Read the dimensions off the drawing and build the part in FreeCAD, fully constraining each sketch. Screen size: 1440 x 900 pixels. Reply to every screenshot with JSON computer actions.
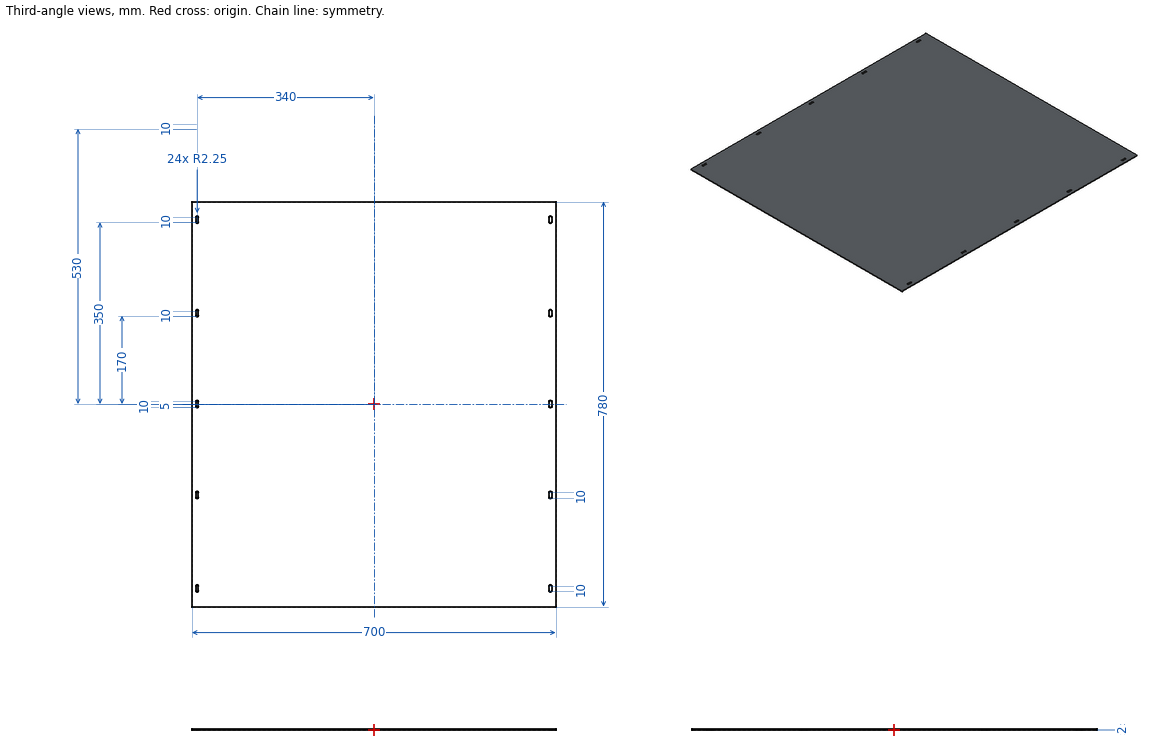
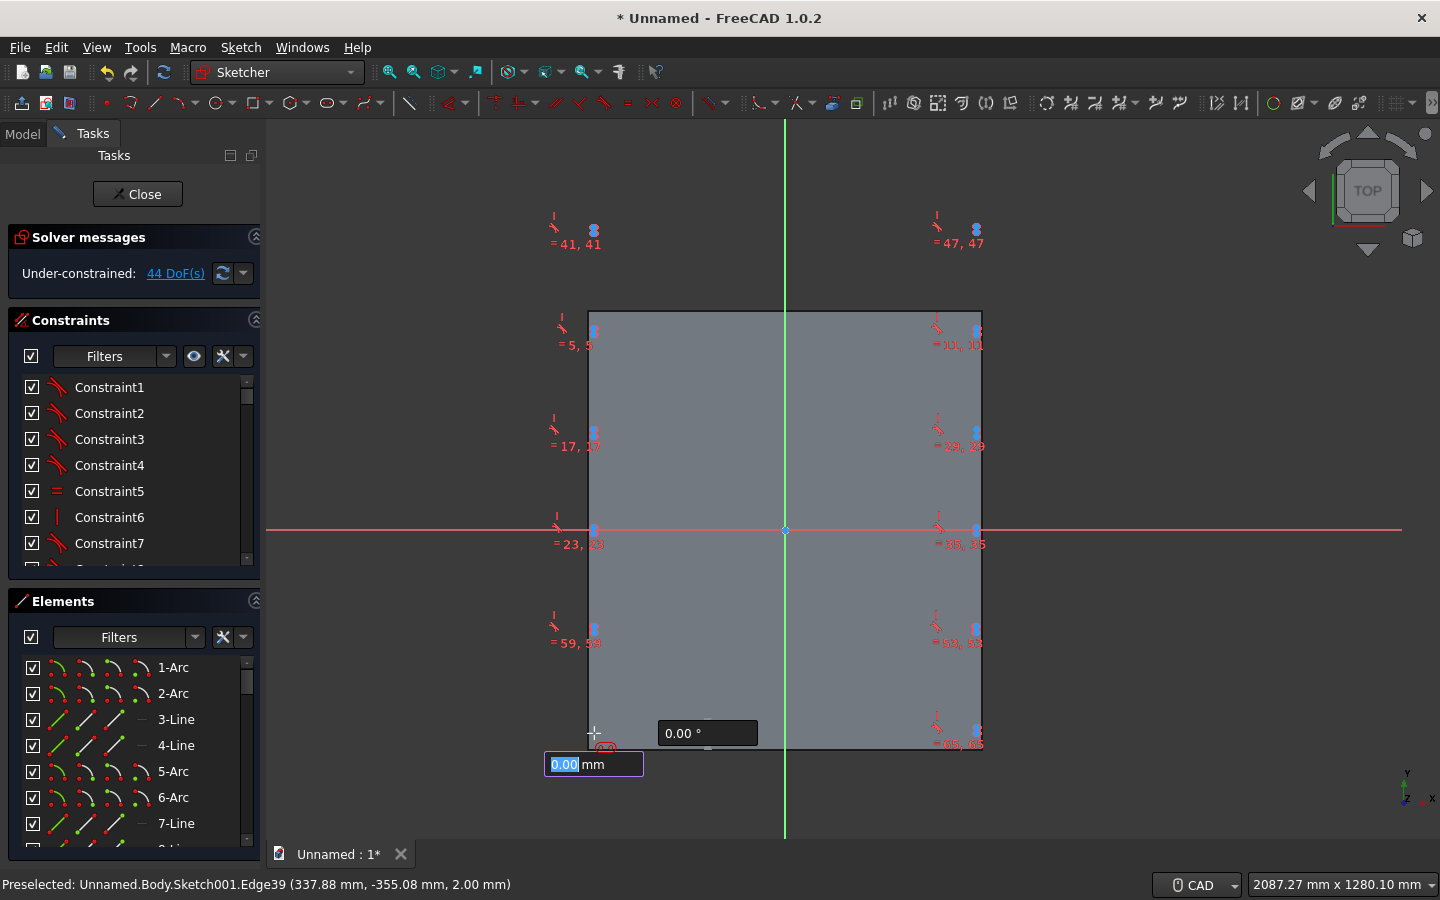
{"action": "scroll", "coordinate": [594, 727], "scroll_direction": "up", "scroll_amount": 6}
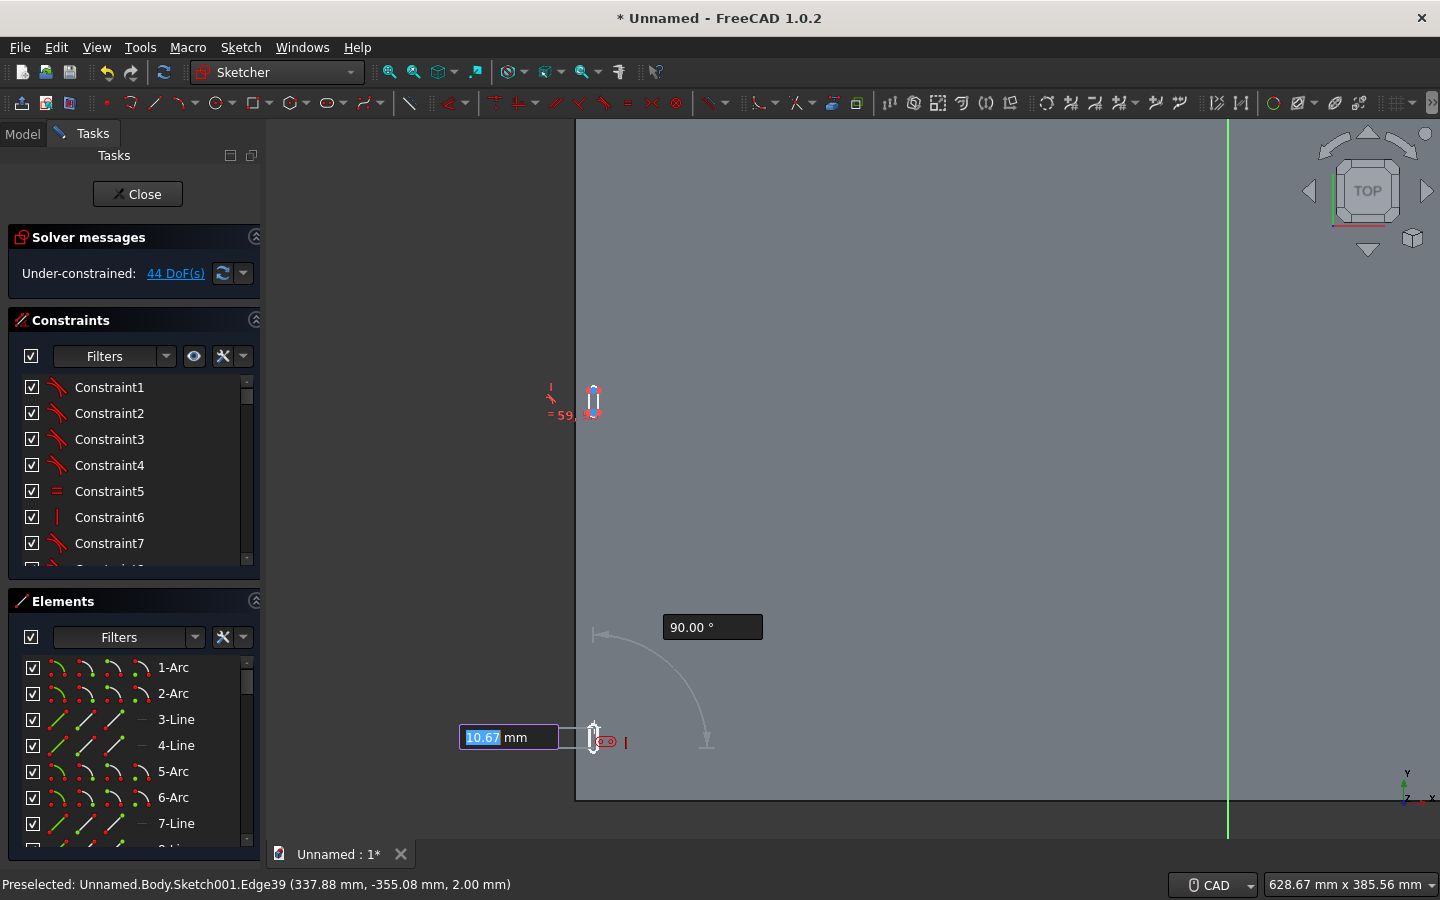
{"action": "left_click", "coordinate": [593, 726]}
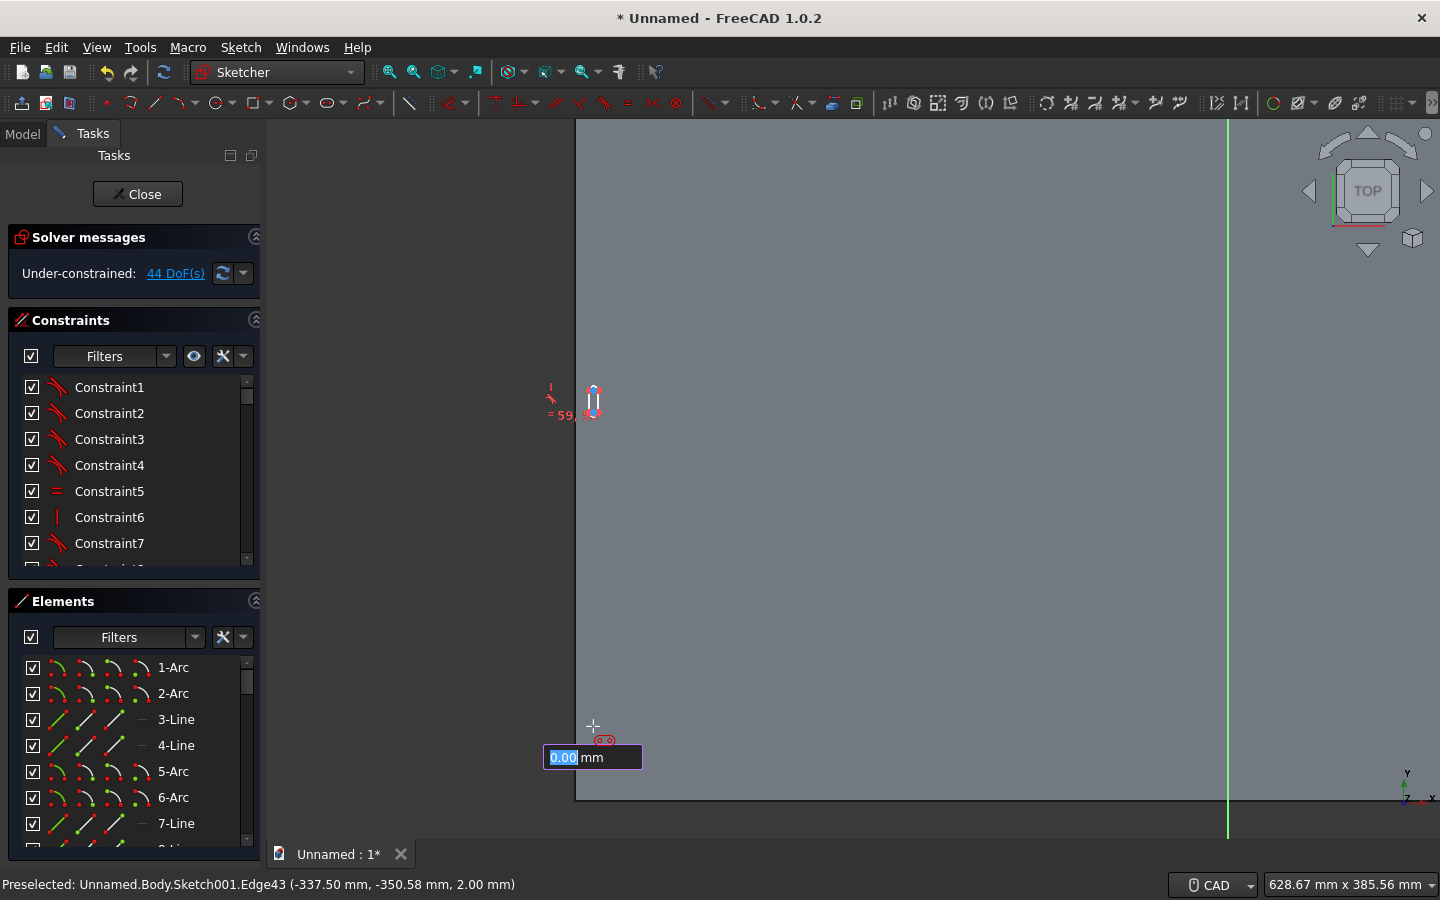
{"action": "scroll", "coordinate": [598, 735], "scroll_direction": "up", "scroll_amount": 7}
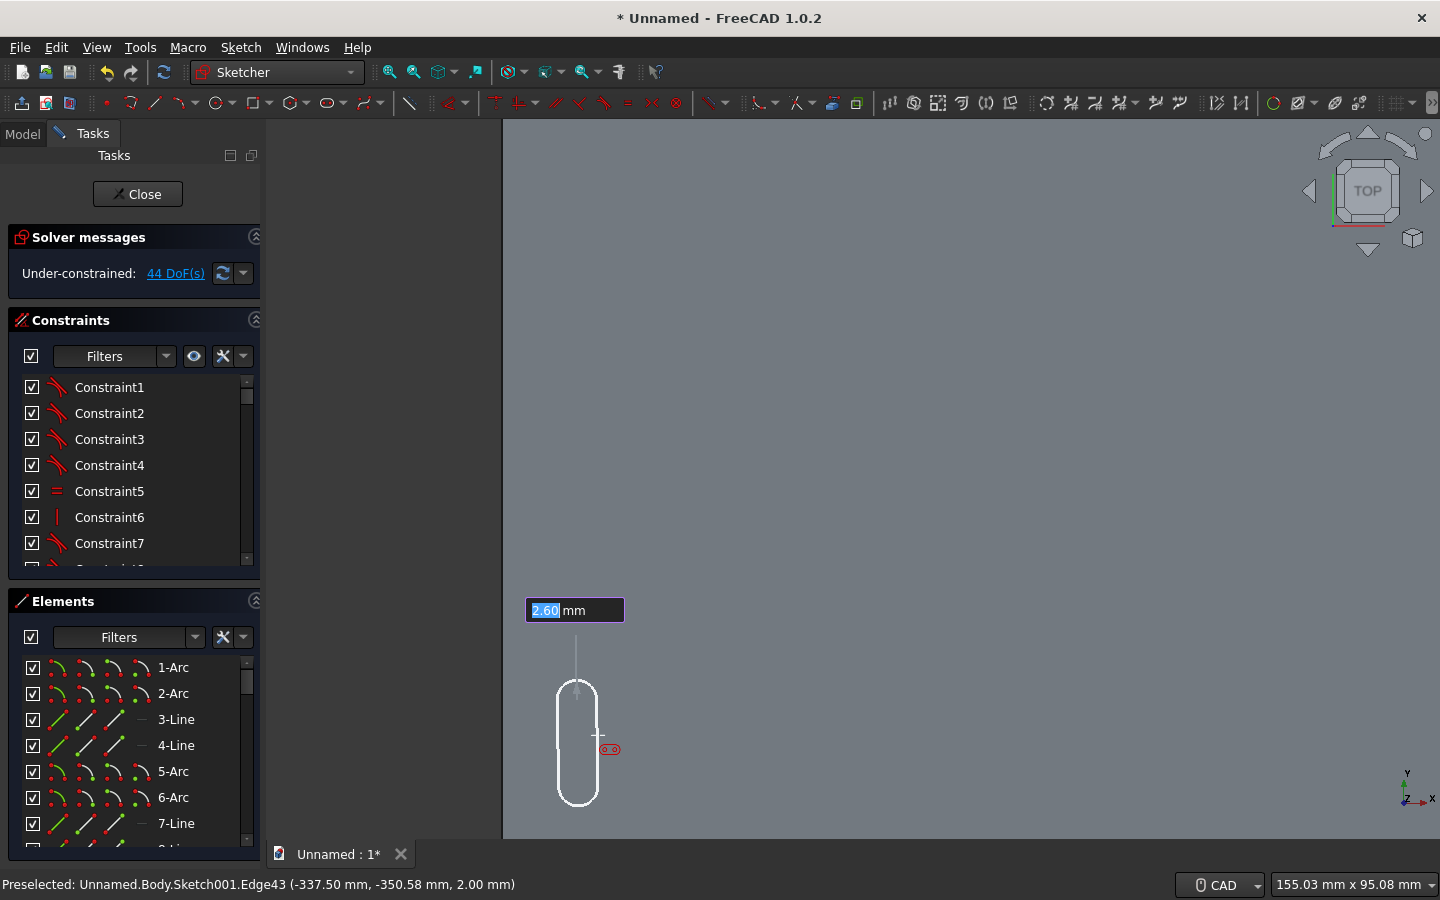
{"action": "left_click", "coordinate": [595, 734]}
{"action": "key", "text": "Escape"}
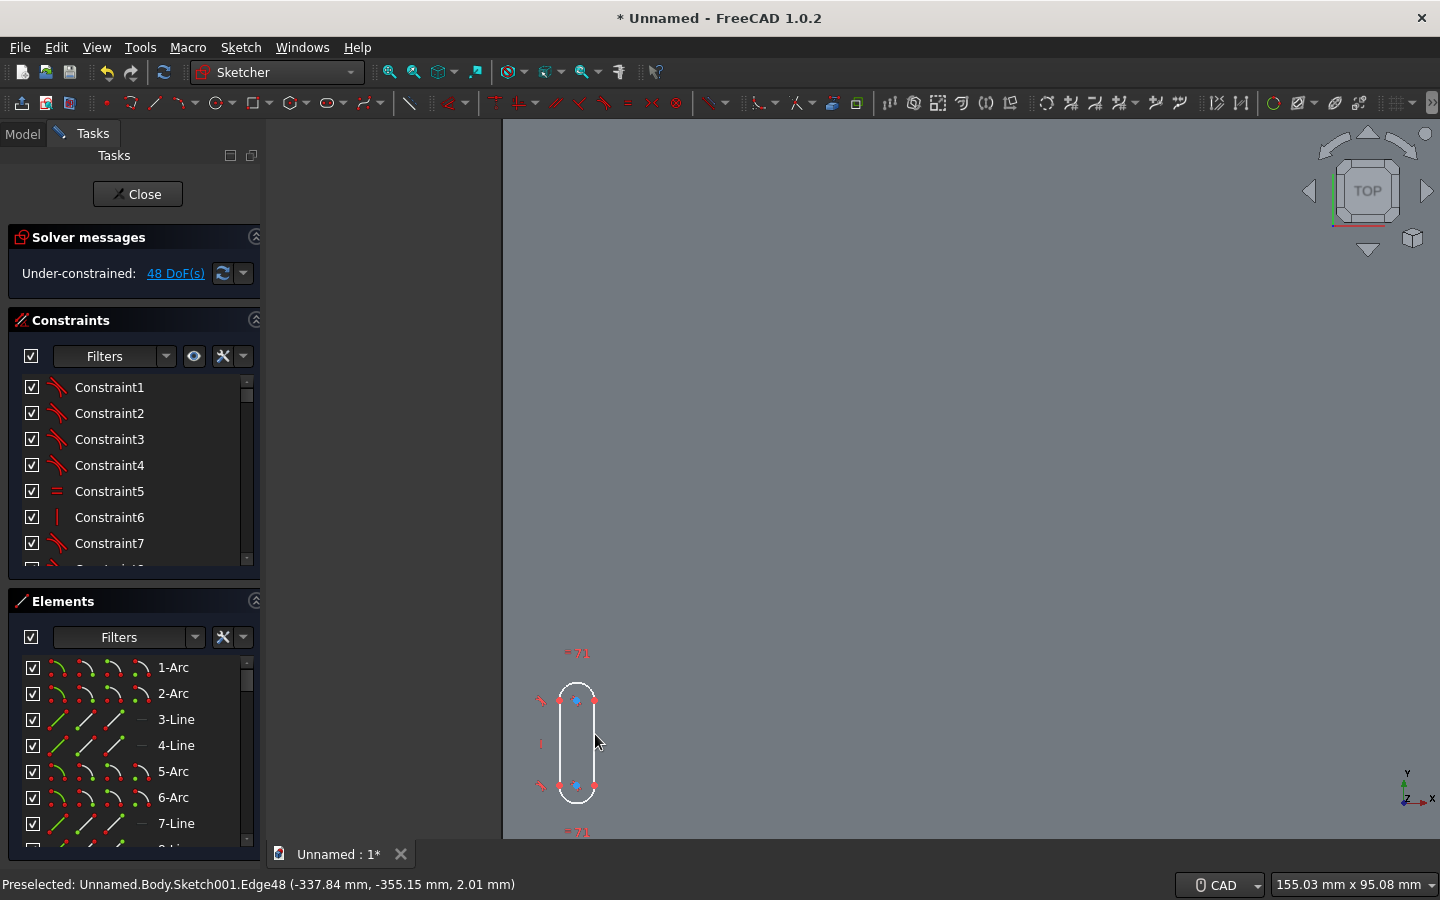
{"action": "scroll", "coordinate": [594, 729], "scroll_direction": "down", "scroll_amount": 13}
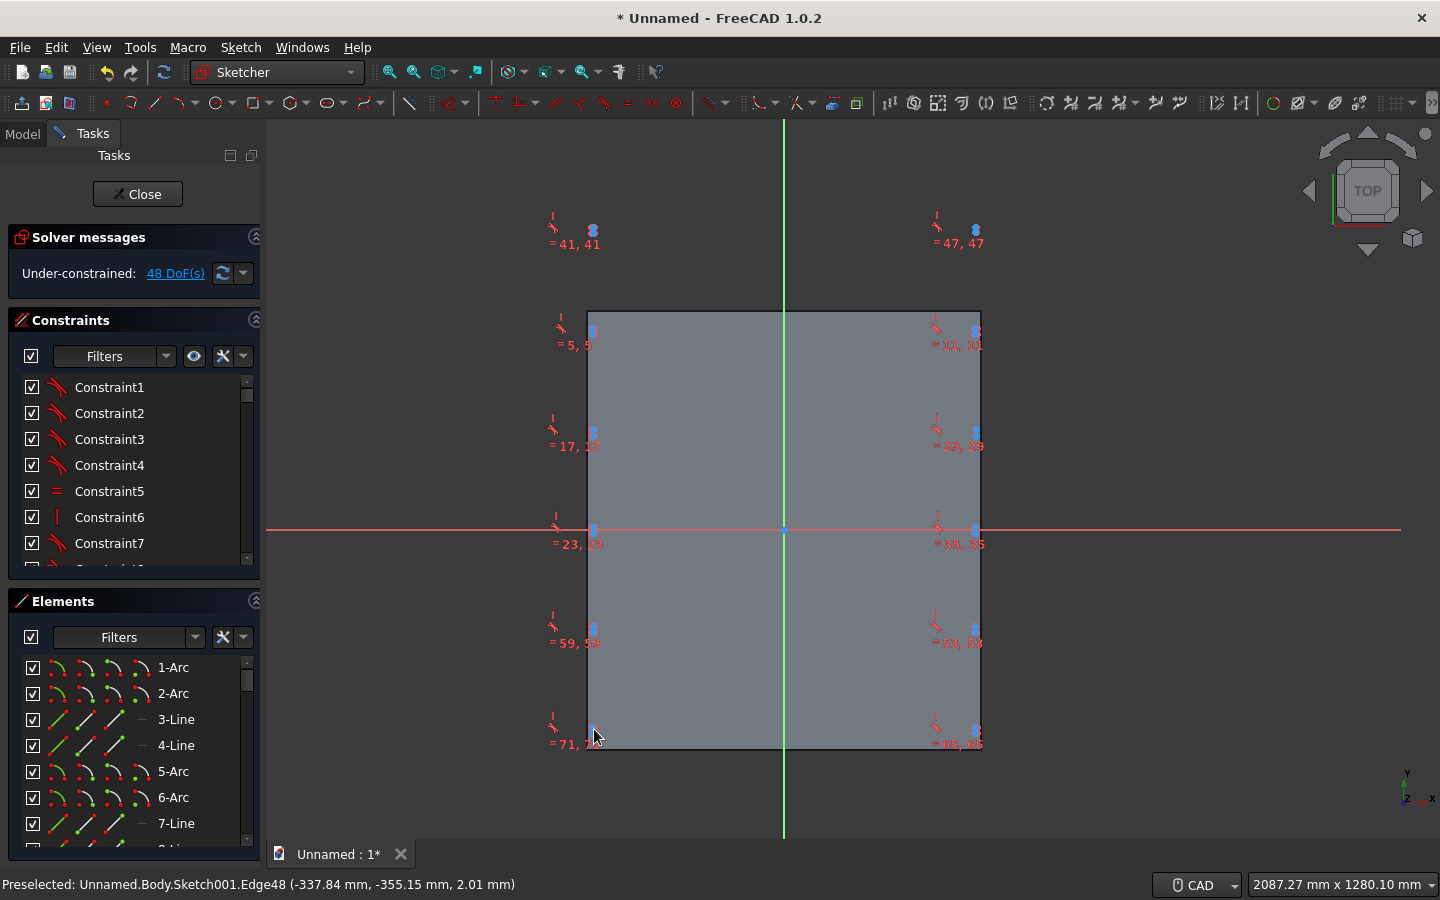
{"action": "scroll", "coordinate": [592, 336], "scroll_direction": "up", "scroll_amount": 12}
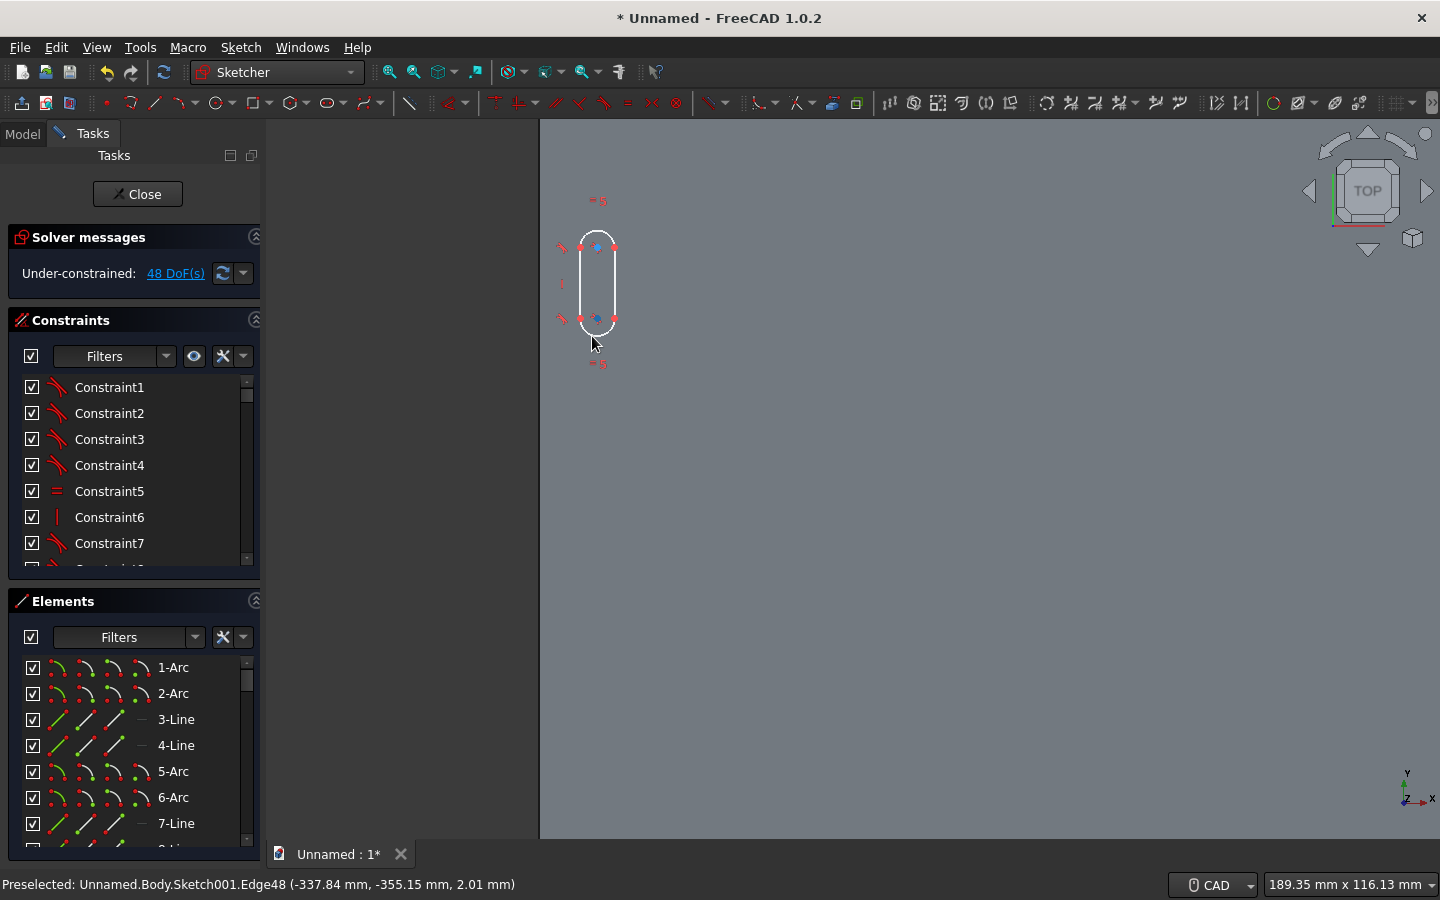
{"action": "left_click", "coordinate": [587, 333]}